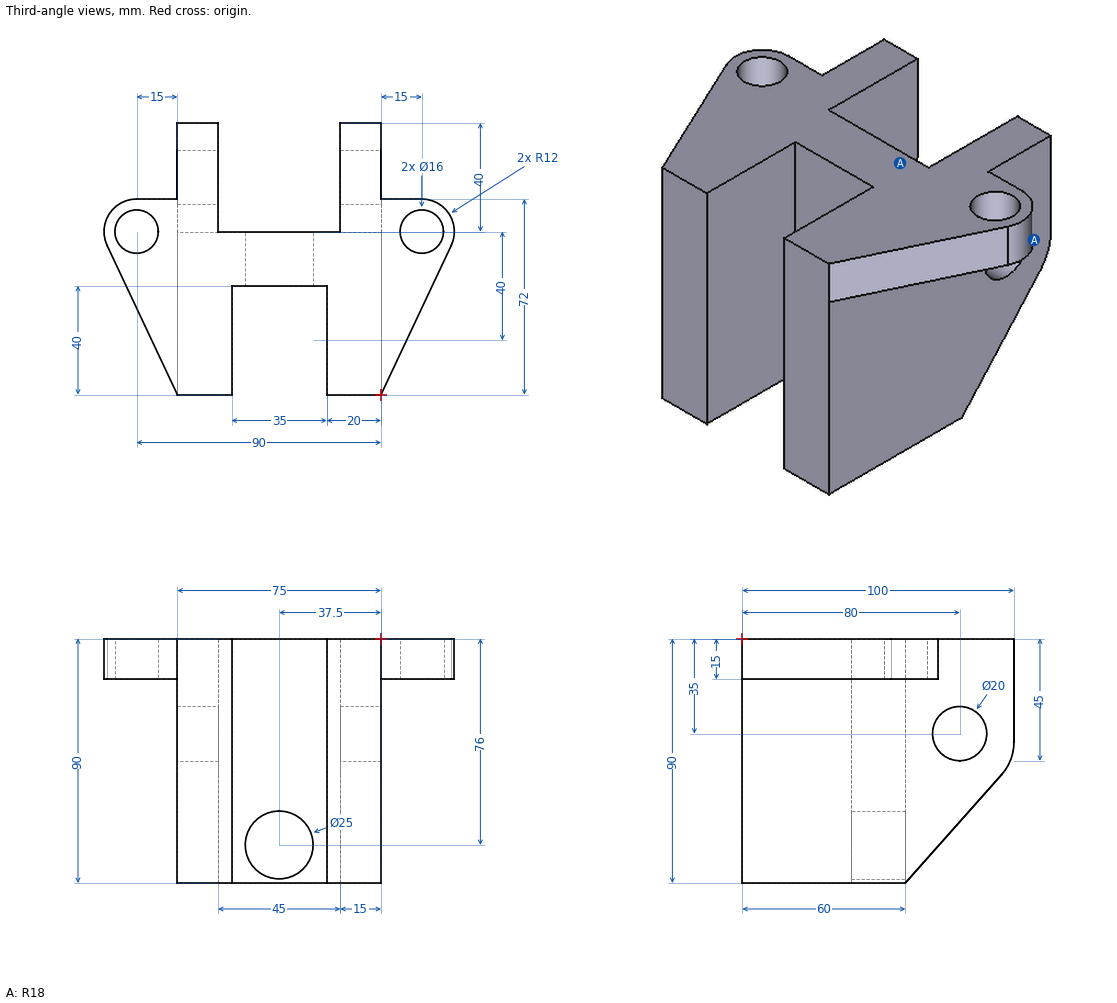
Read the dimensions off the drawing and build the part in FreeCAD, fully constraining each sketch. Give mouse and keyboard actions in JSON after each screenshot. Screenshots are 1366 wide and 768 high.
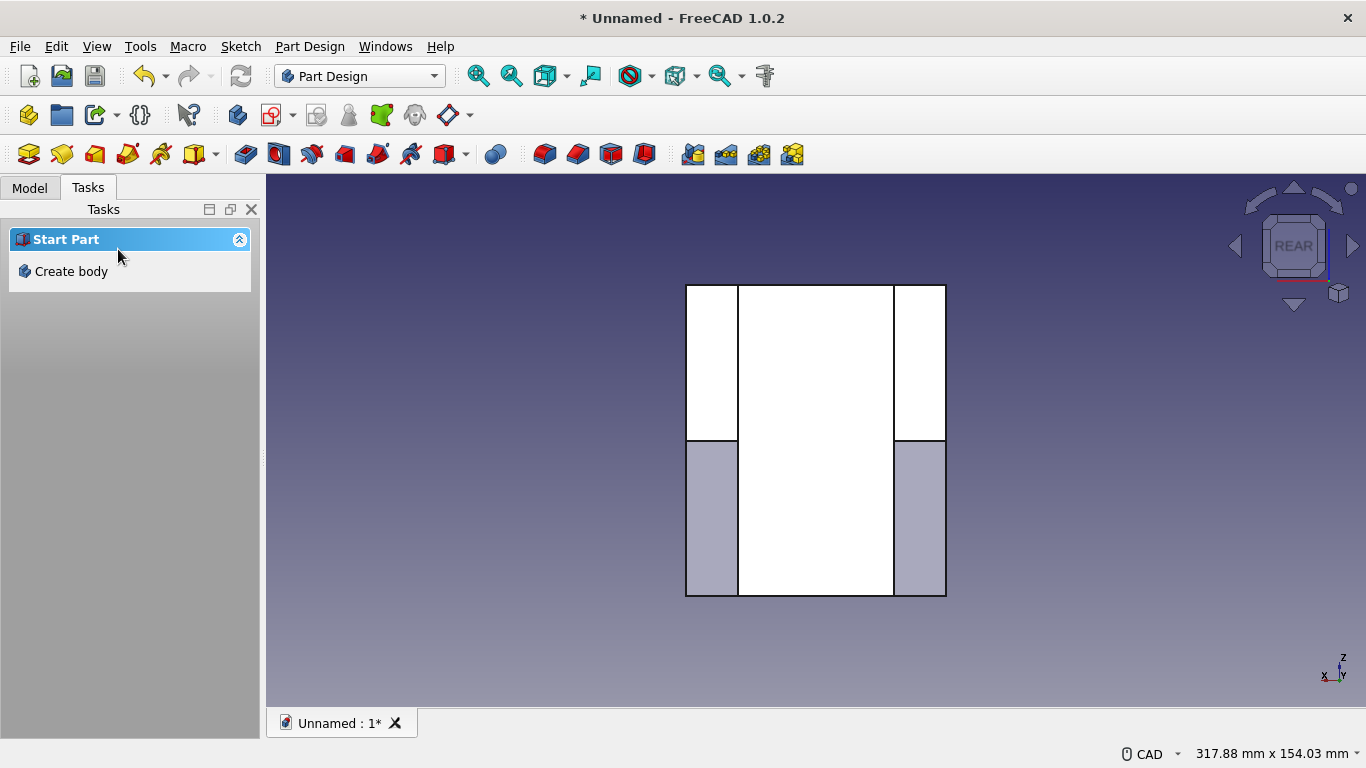
{"action": "left_click", "coordinate": [712, 439]}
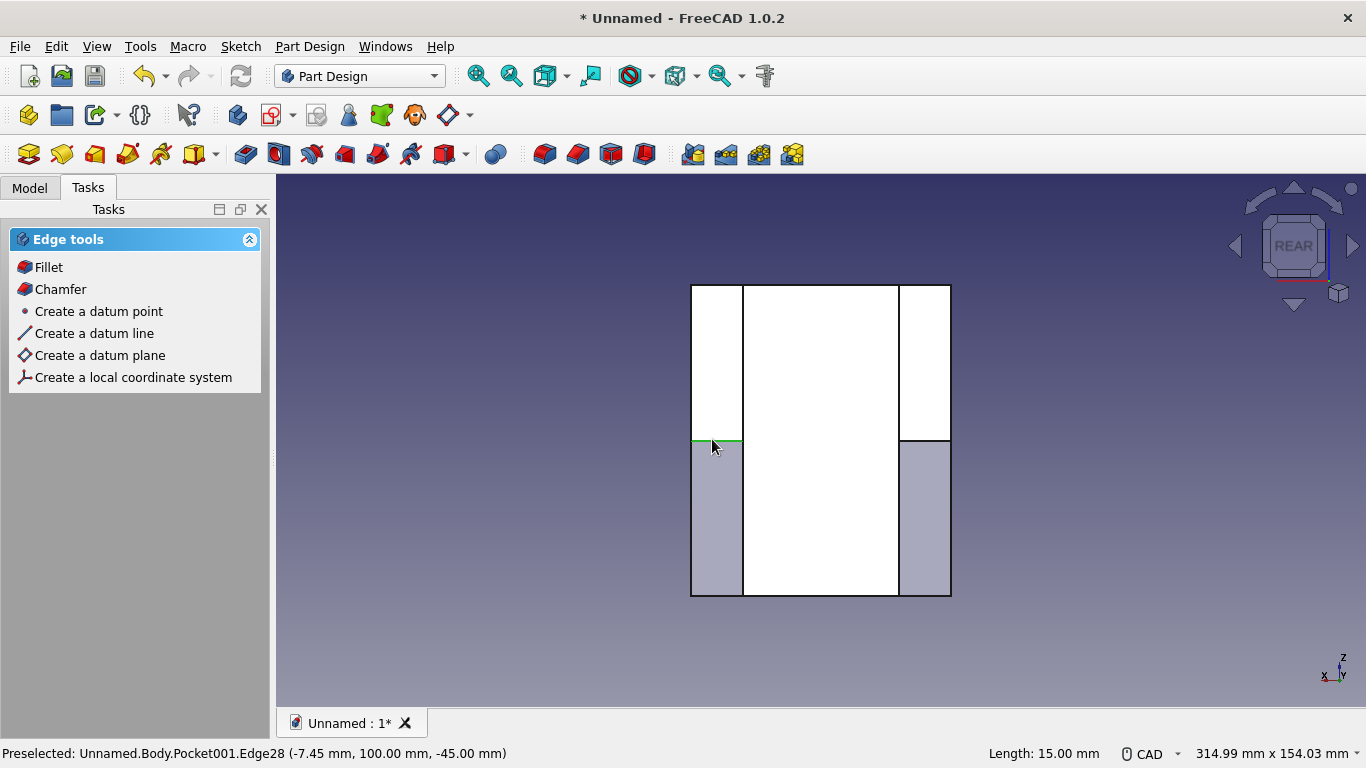
{"action": "left_click", "coordinate": [925, 439], "text": "ctrl"}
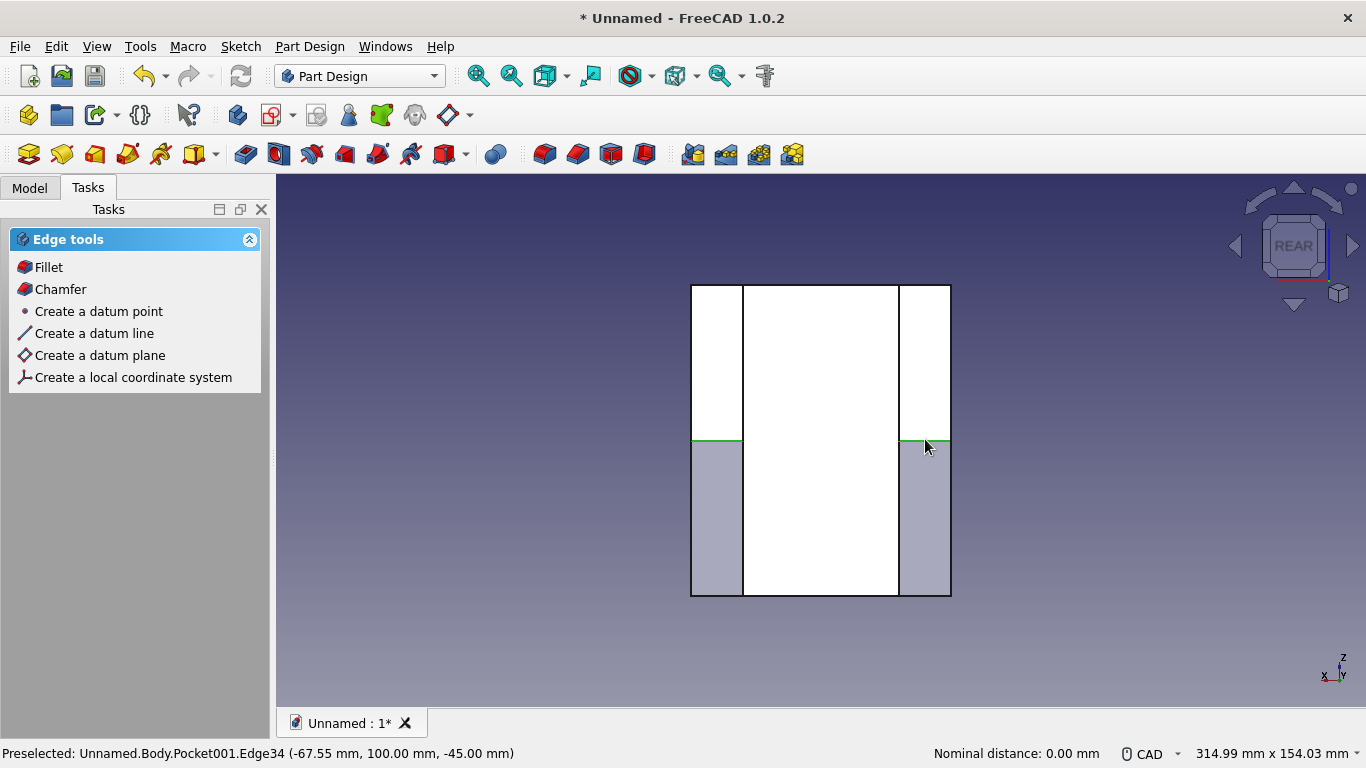
{"action": "left_click", "coordinate": [545, 154]}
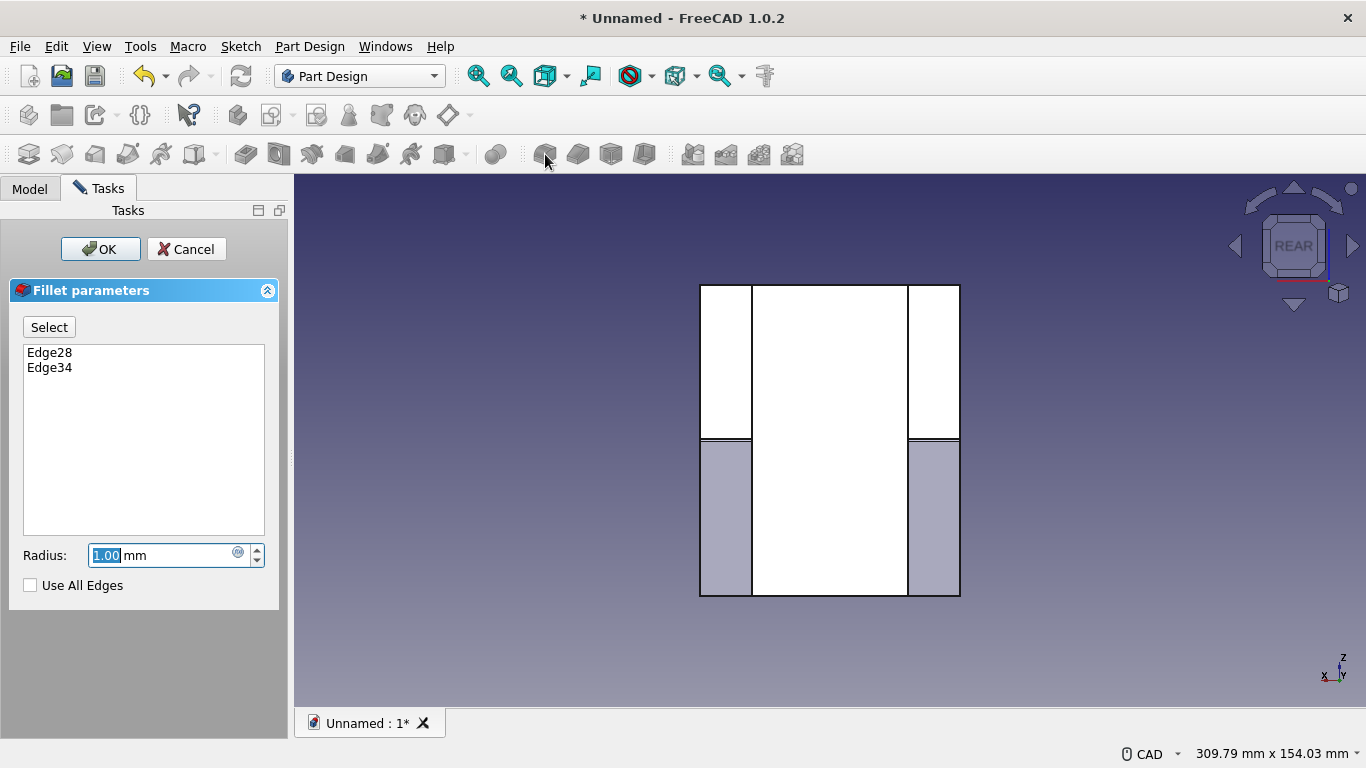
{"action": "type", "text": "18"}
{"action": "key", "text": "Tab"}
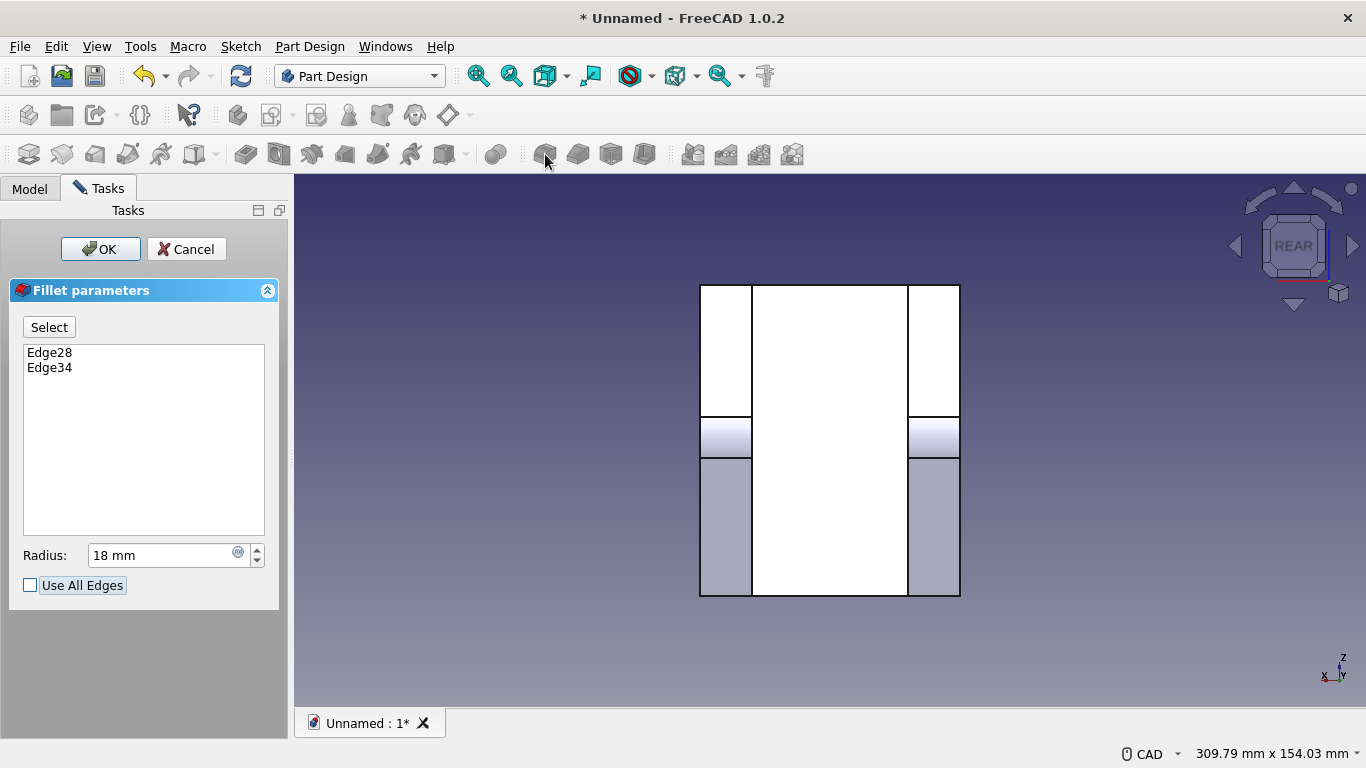
{"action": "left_click", "coordinate": [101, 249]}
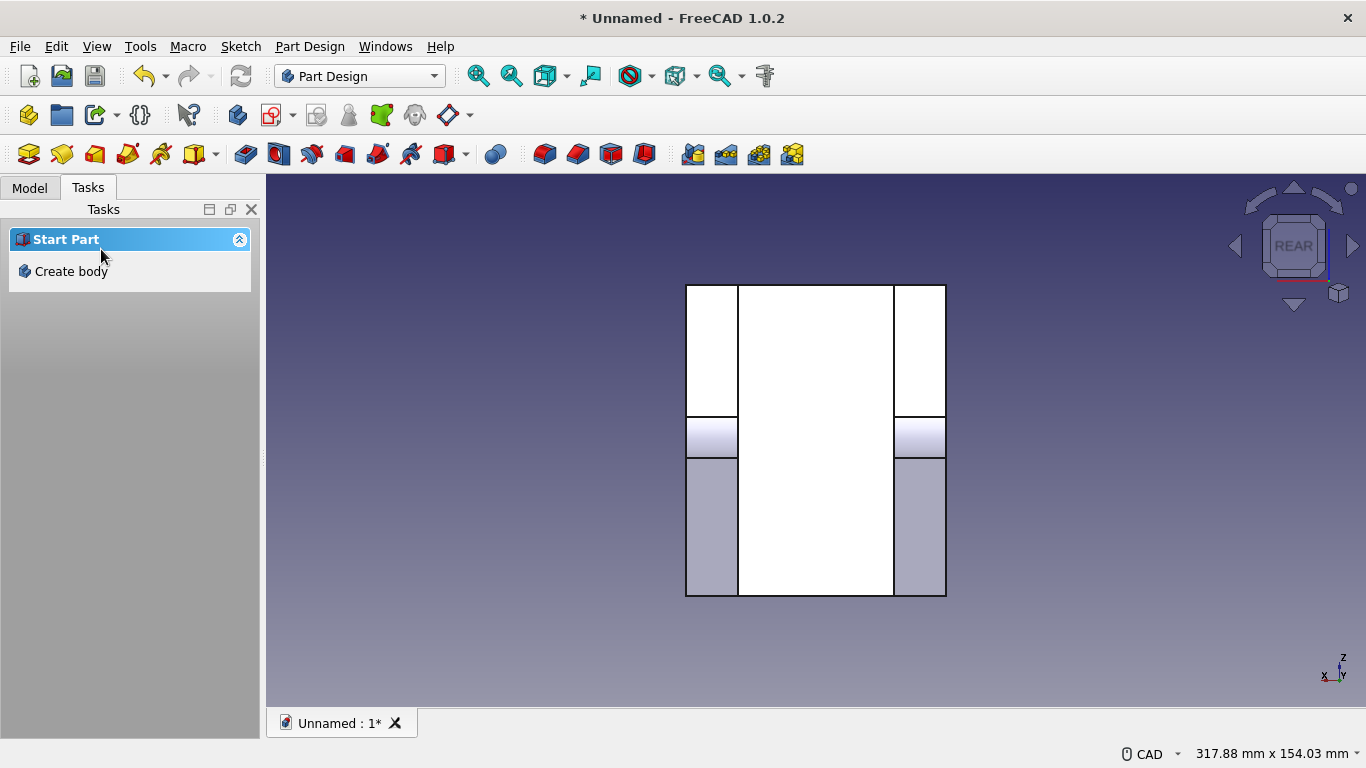
{"action": "key", "text": "0"}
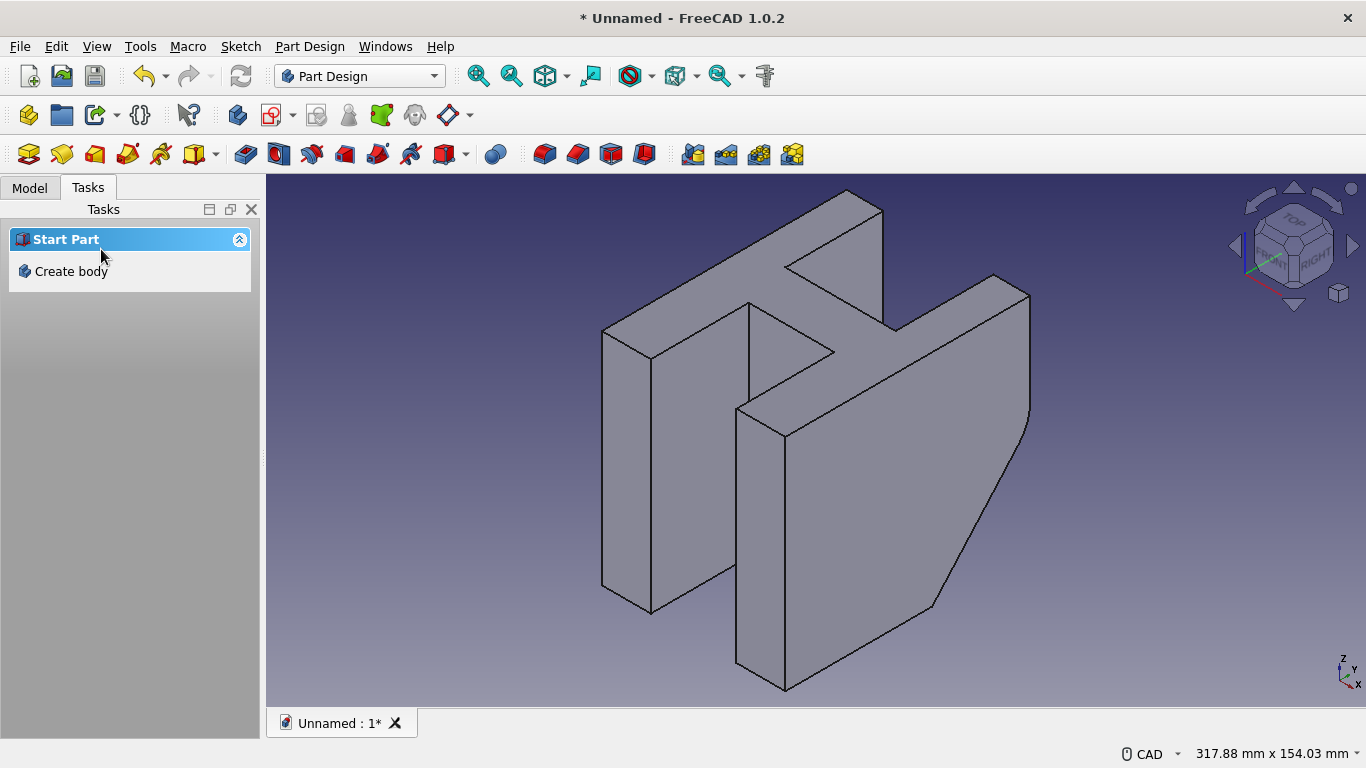
{"action": "left_click", "coordinate": [908, 492]}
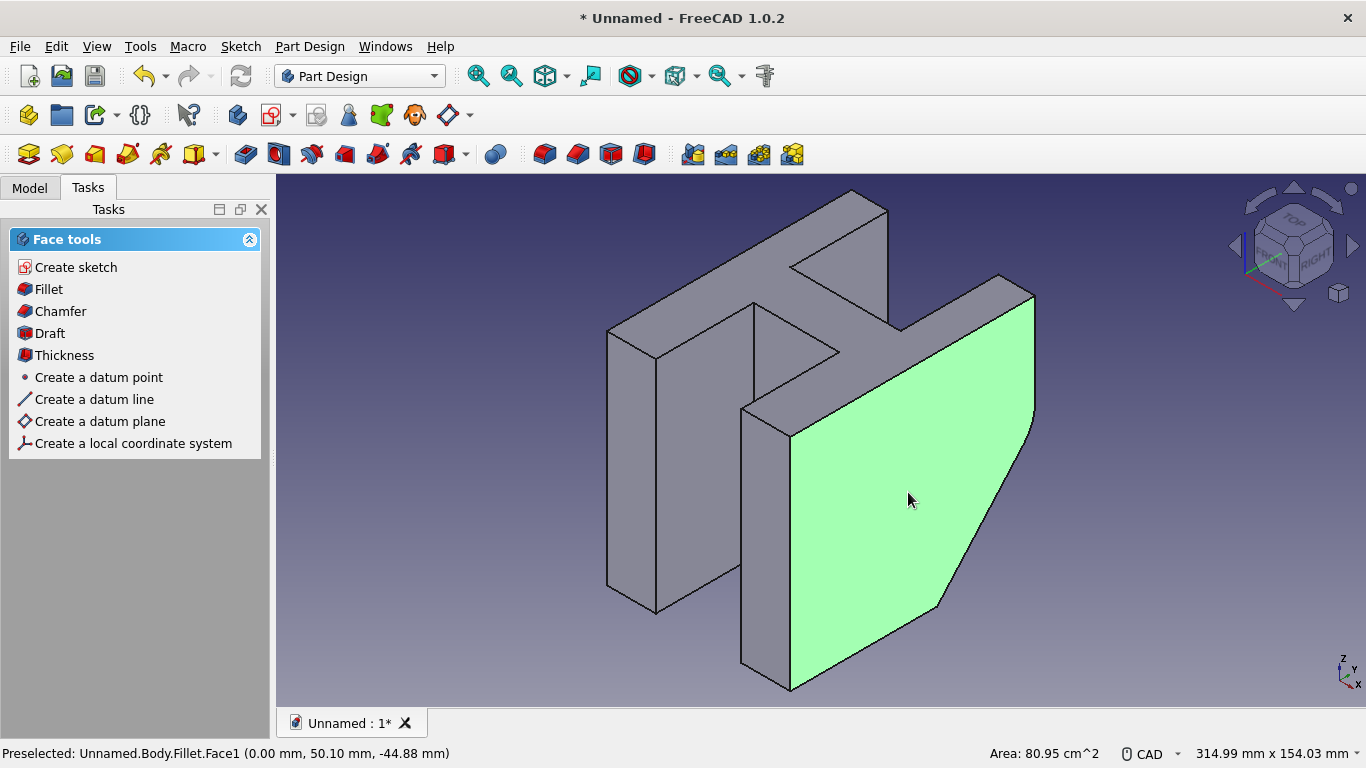
{"action": "left_click", "coordinate": [270, 116]}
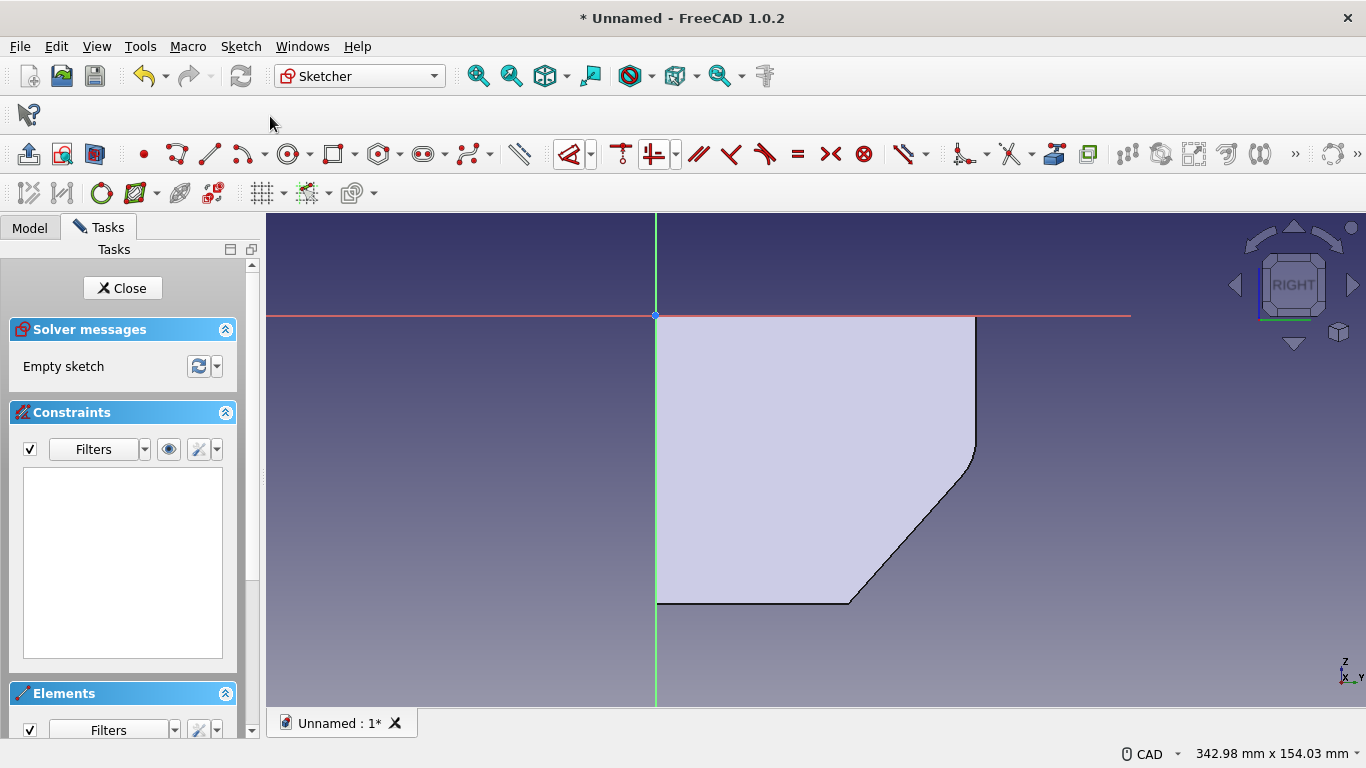
{"action": "scroll", "coordinate": [954, 420], "scroll_direction": "up", "scroll_amount": 8}